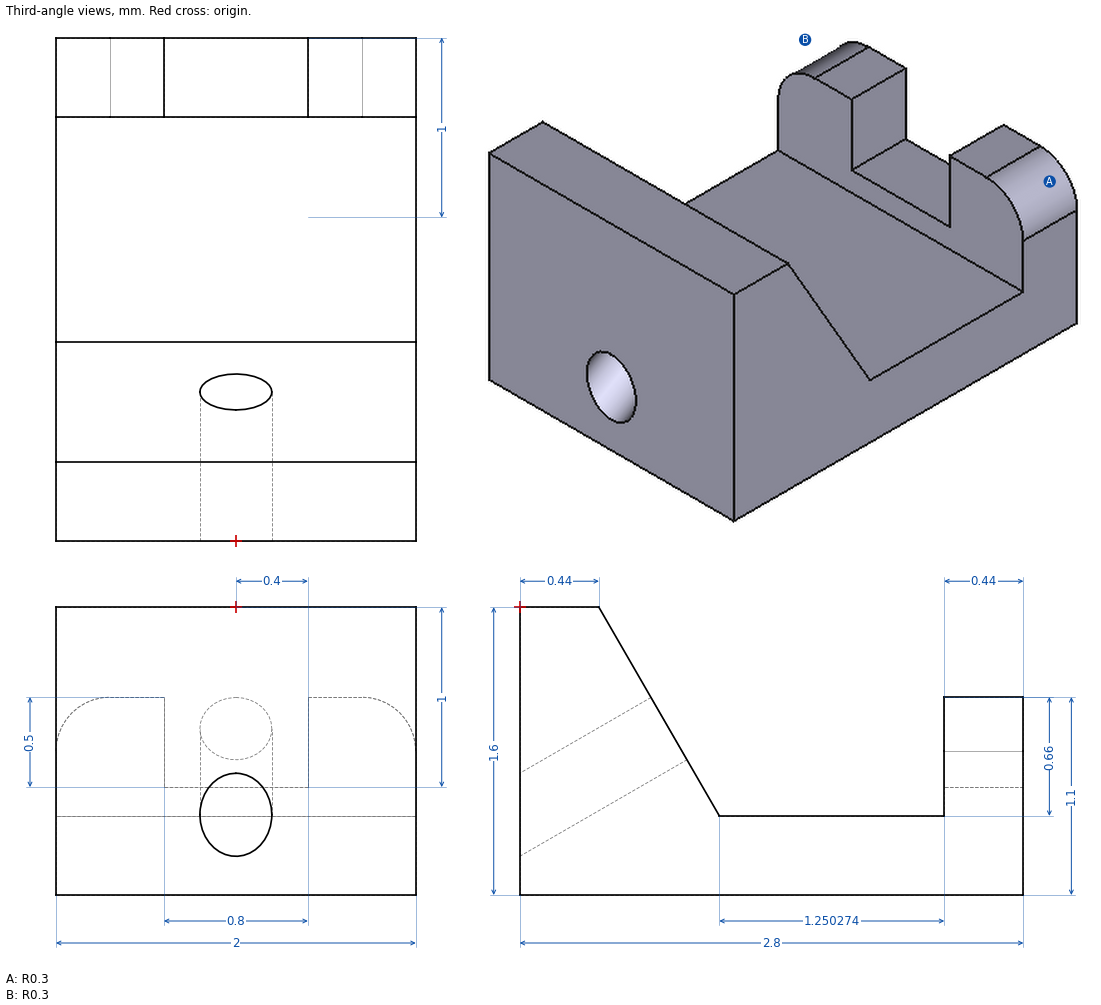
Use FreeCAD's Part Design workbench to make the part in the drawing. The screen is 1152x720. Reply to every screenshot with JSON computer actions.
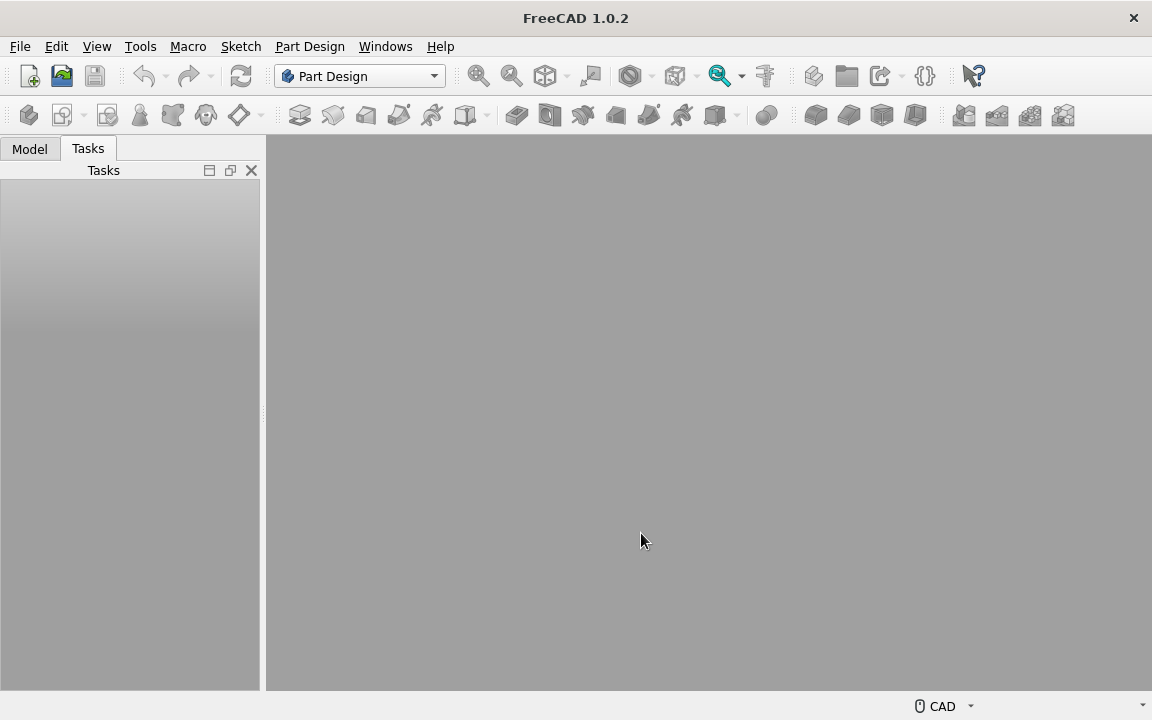
{"action": "key", "text": "ctrl+n"}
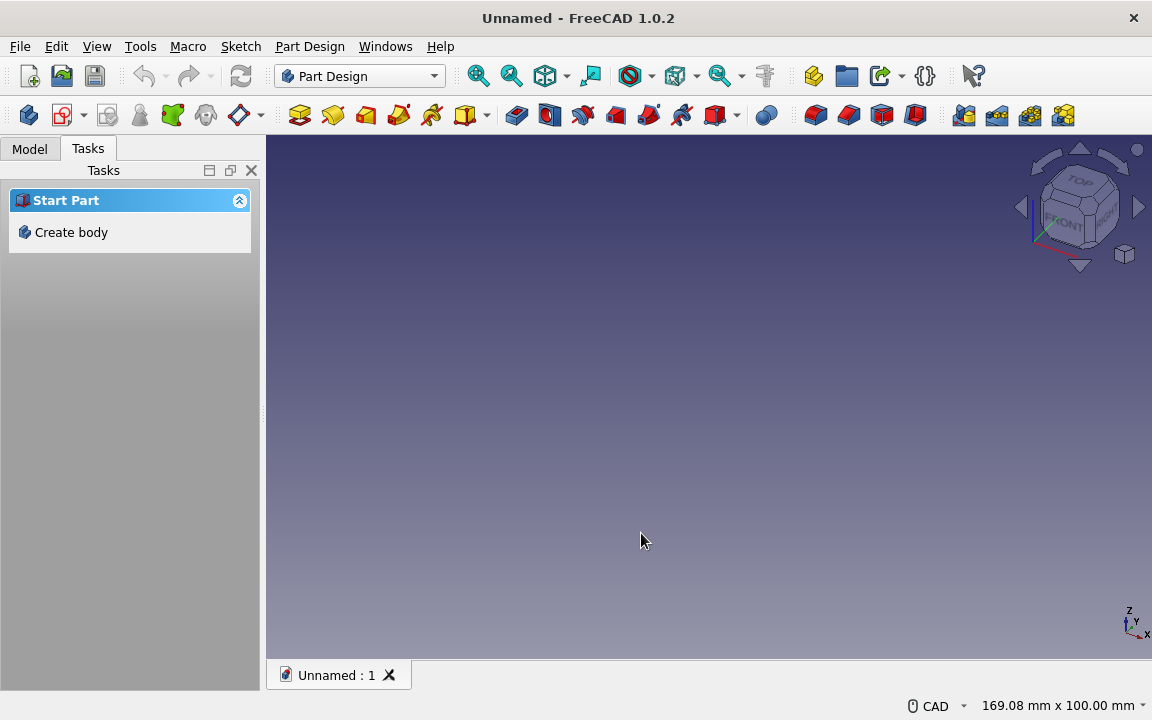
{"action": "left_click", "coordinate": [62, 116]}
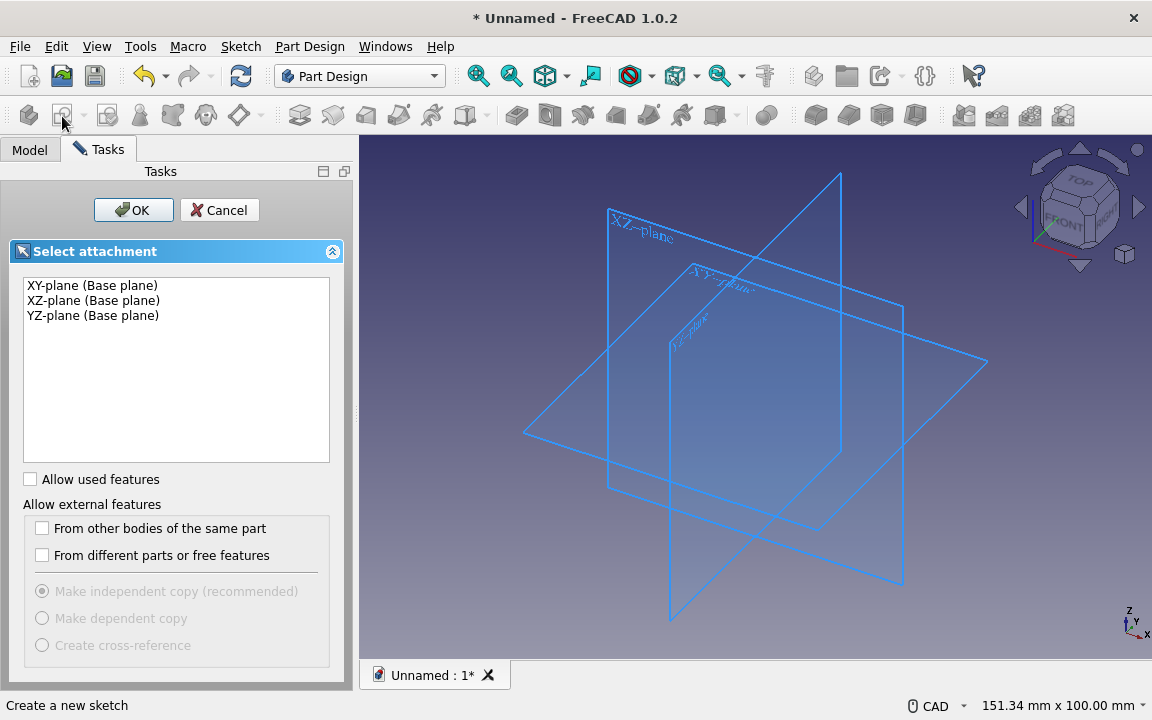
{"action": "left_click", "coordinate": [84, 316]}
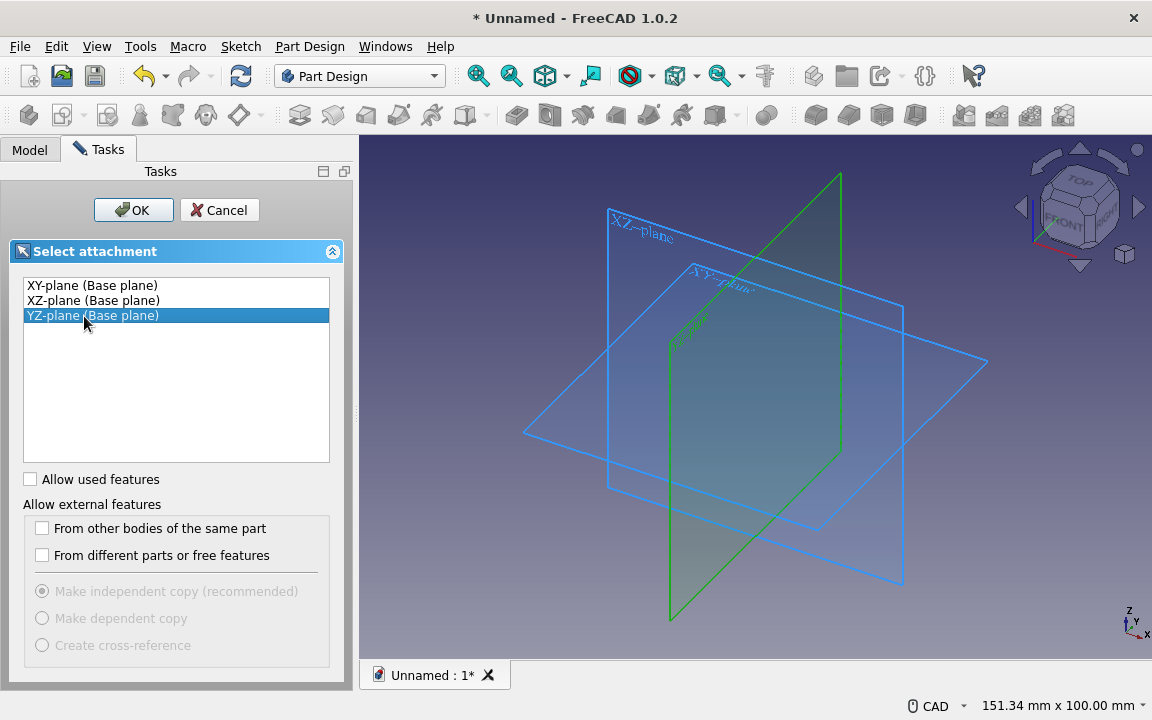
{"action": "left_click", "coordinate": [134, 210]}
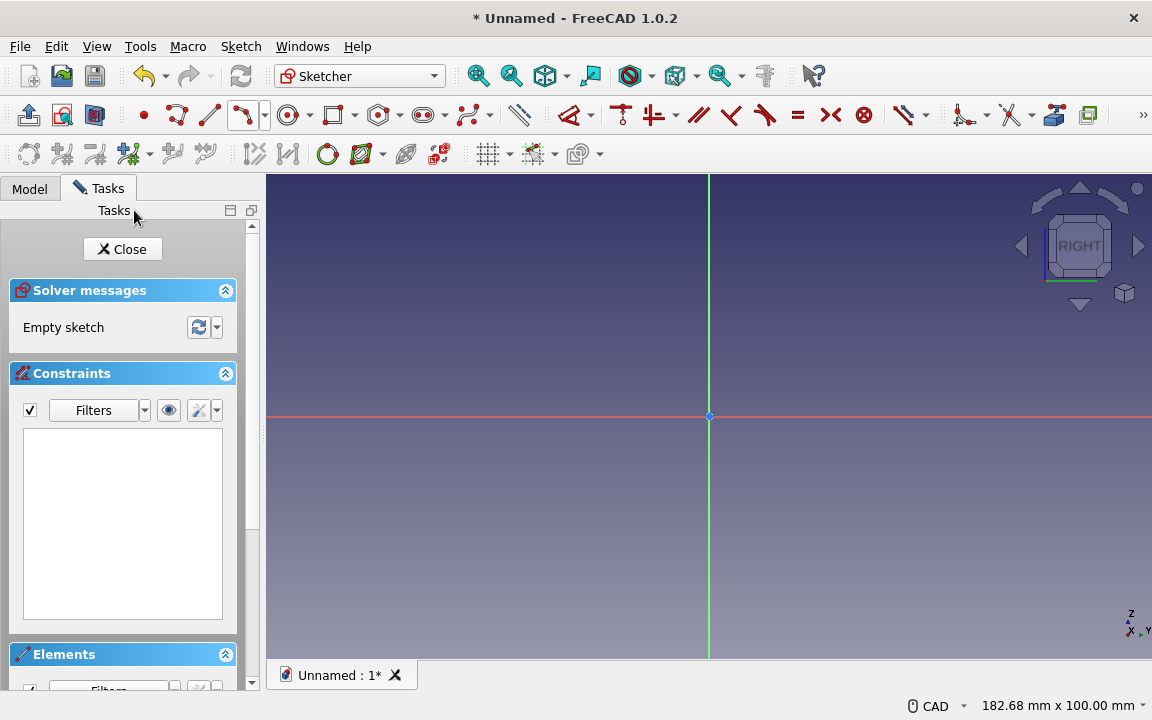
{"action": "scroll", "coordinate": [720, 421], "scroll_direction": "up", "scroll_amount": 15}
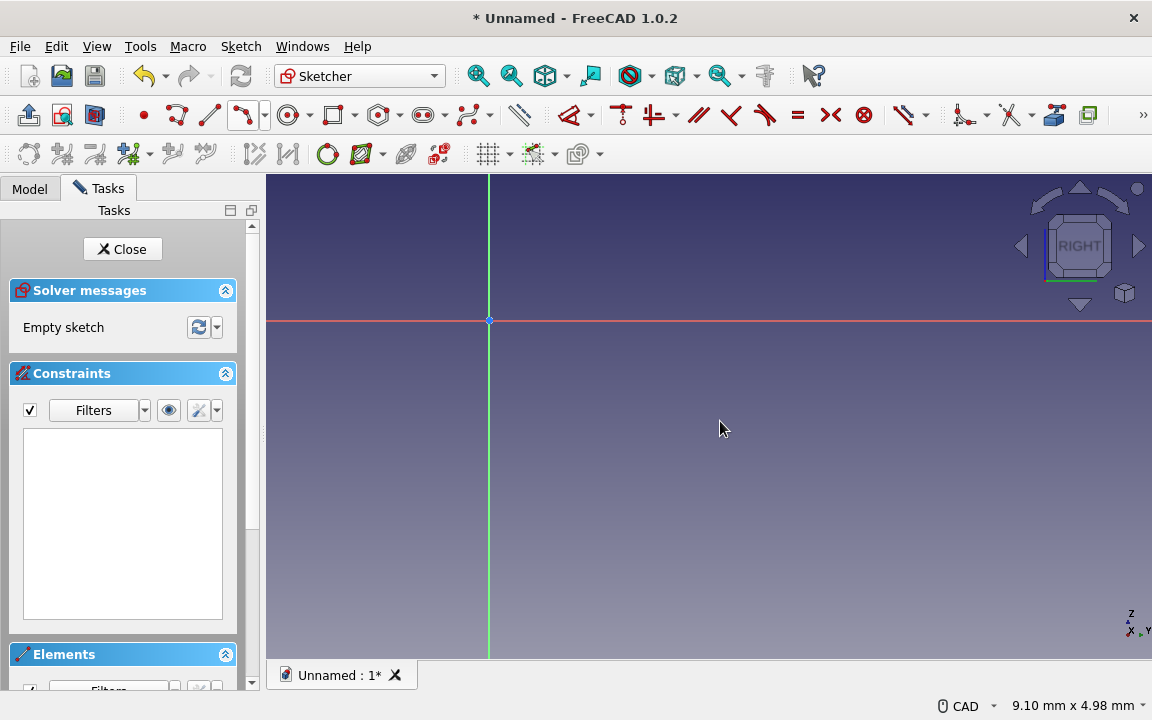
{"action": "scroll", "coordinate": [608, 377], "scroll_direction": "up", "scroll_amount": 3}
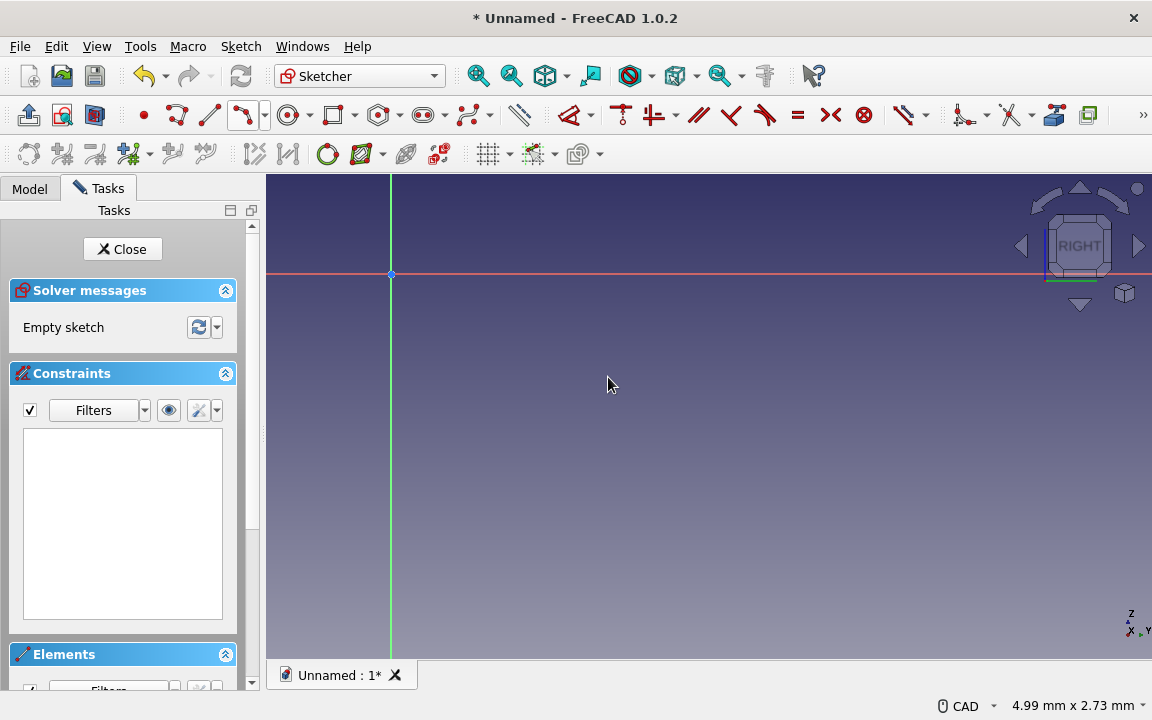
{"action": "key", "text": "g m"}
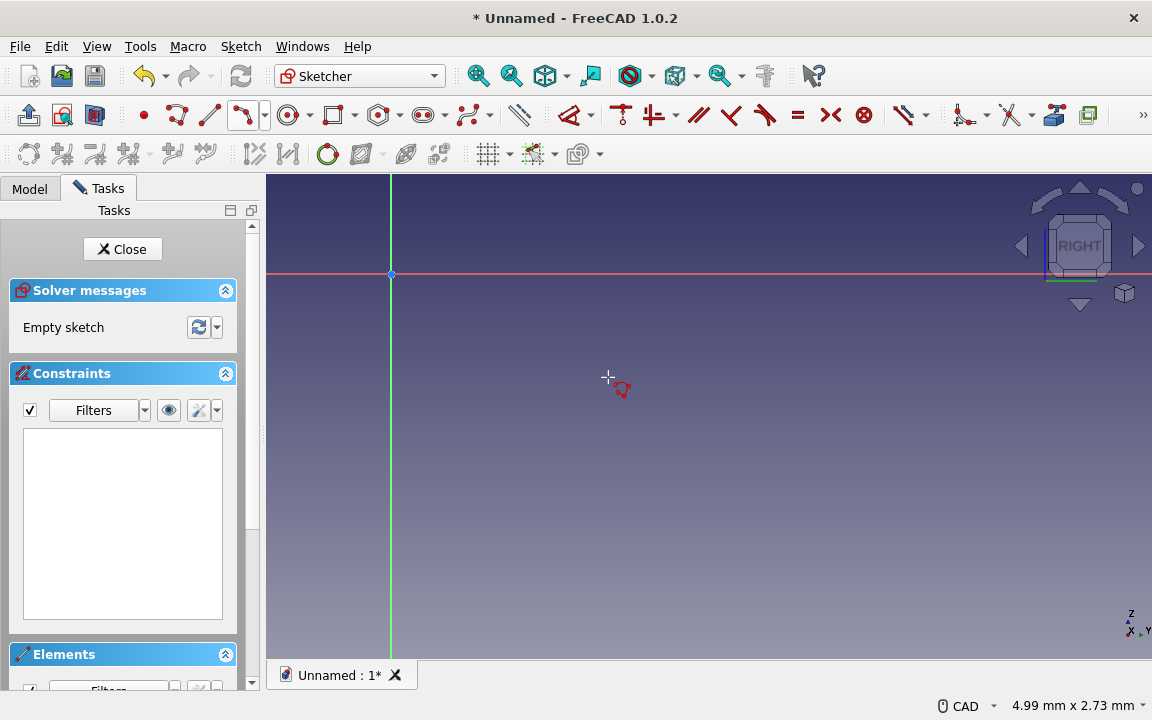
{"action": "left_click", "coordinate": [391, 274]}
{"action": "left_click", "coordinate": [400, 558]}
{"action": "left_click", "coordinate": [888, 558]}
{"action": "left_click", "coordinate": [888, 363]}
{"action": "left_click", "coordinate": [810, 363]}
{"action": "left_click", "coordinate": [810, 480]}
{"action": "left_click", "coordinate": [588, 480]}
{"action": "left_click", "coordinate": [469, 283]}
{"action": "left_click", "coordinate": [391, 274]}
{"action": "key", "text": "Escape"}
{"action": "key", "text": "Escape"}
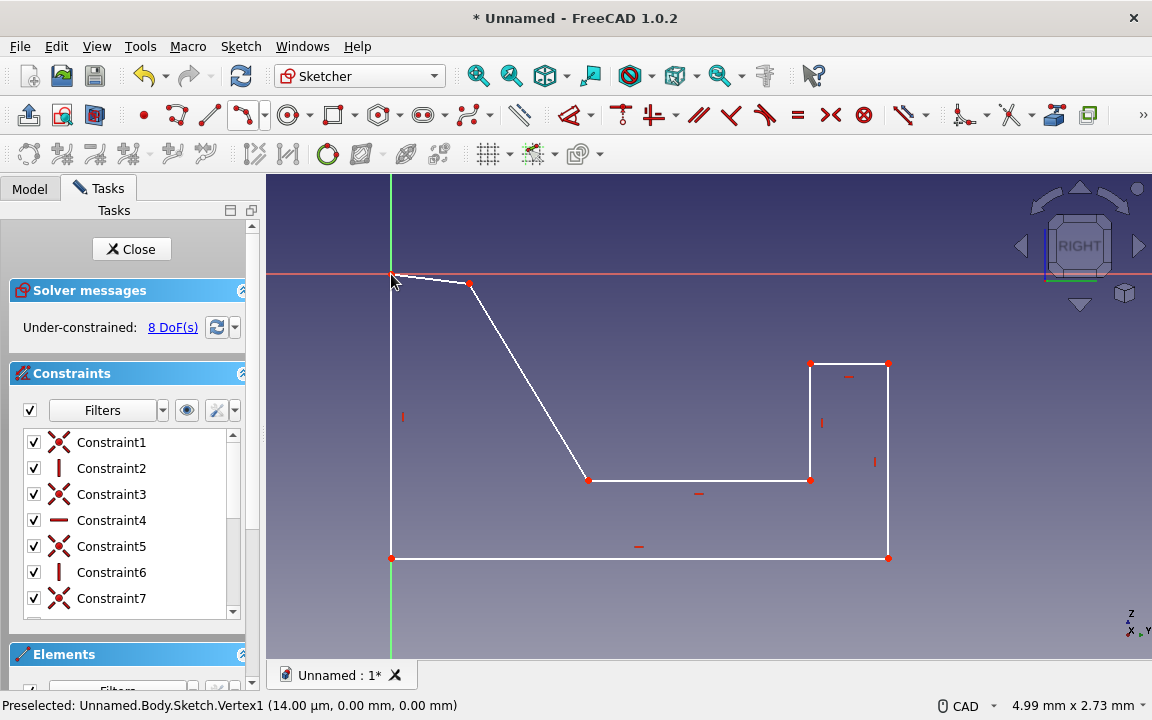
{"action": "left_click", "coordinate": [415, 277]}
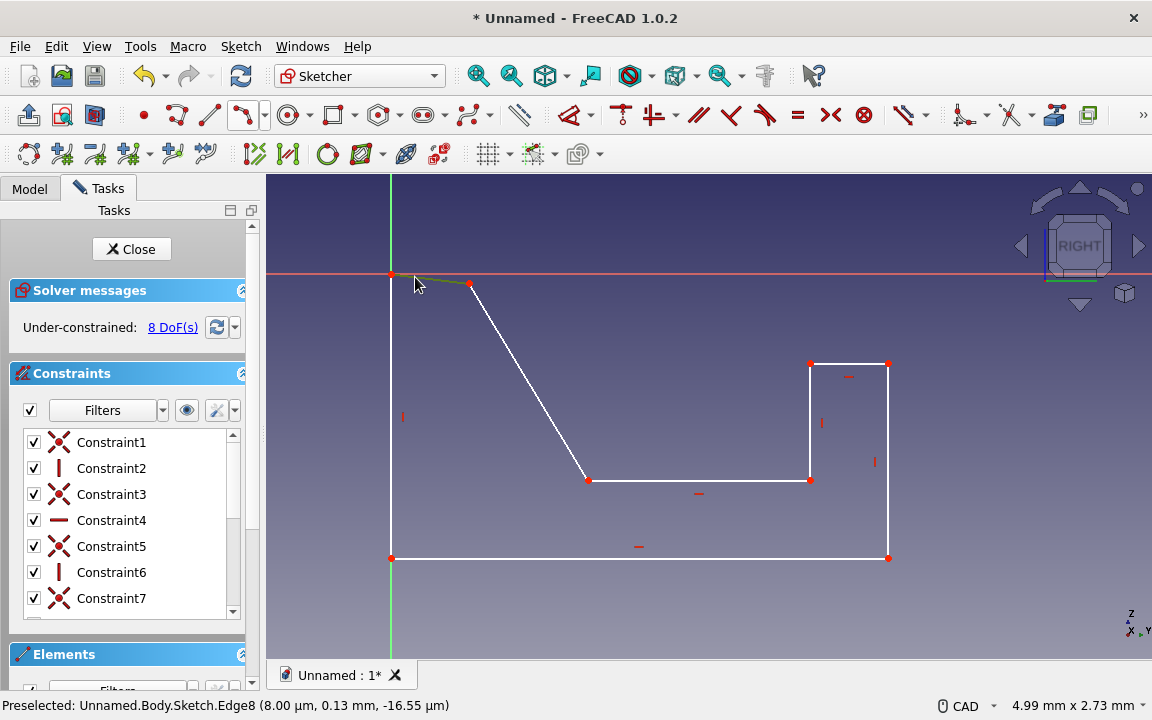
{"action": "key", "text": "h"}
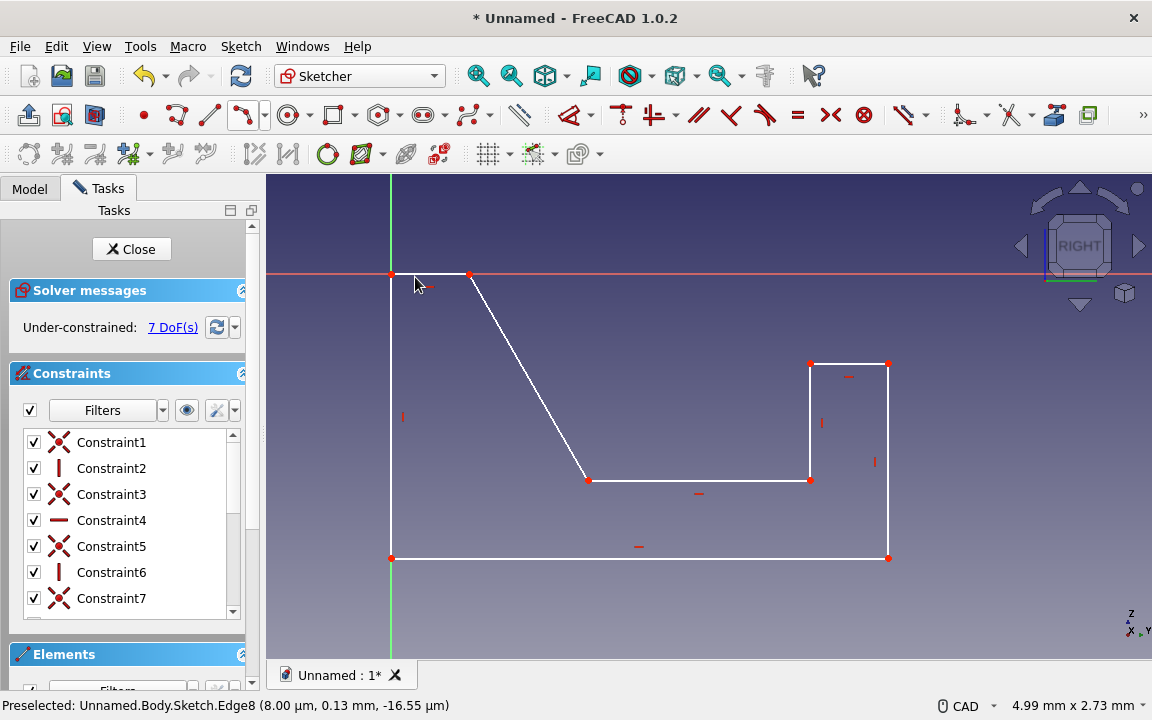
{"action": "left_click", "coordinate": [568, 116]}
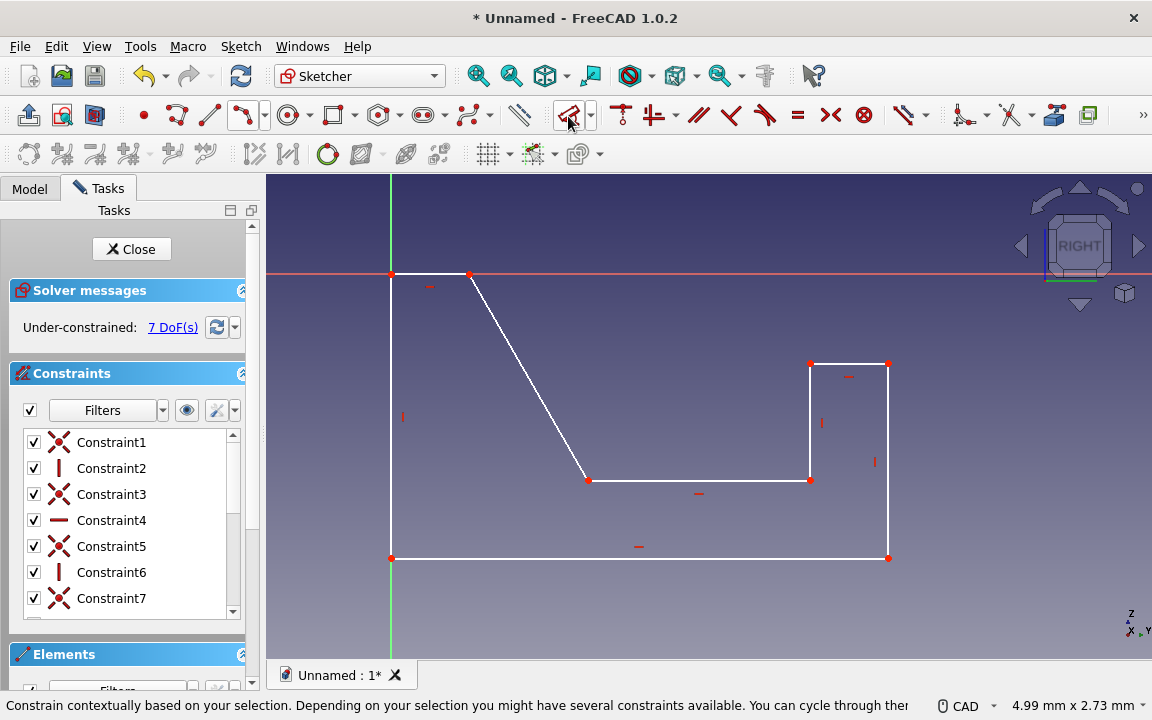
{"action": "left_click", "coordinate": [391, 360]}
{"action": "left_click", "coordinate": [357, 417]}